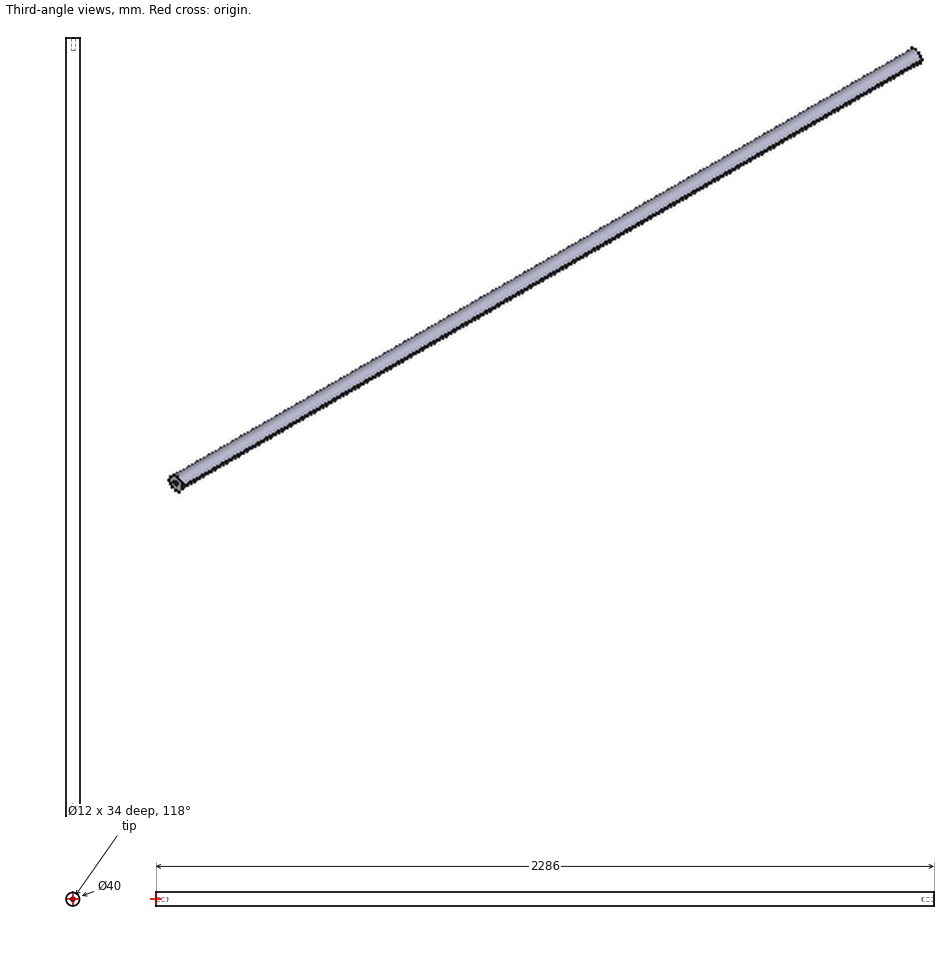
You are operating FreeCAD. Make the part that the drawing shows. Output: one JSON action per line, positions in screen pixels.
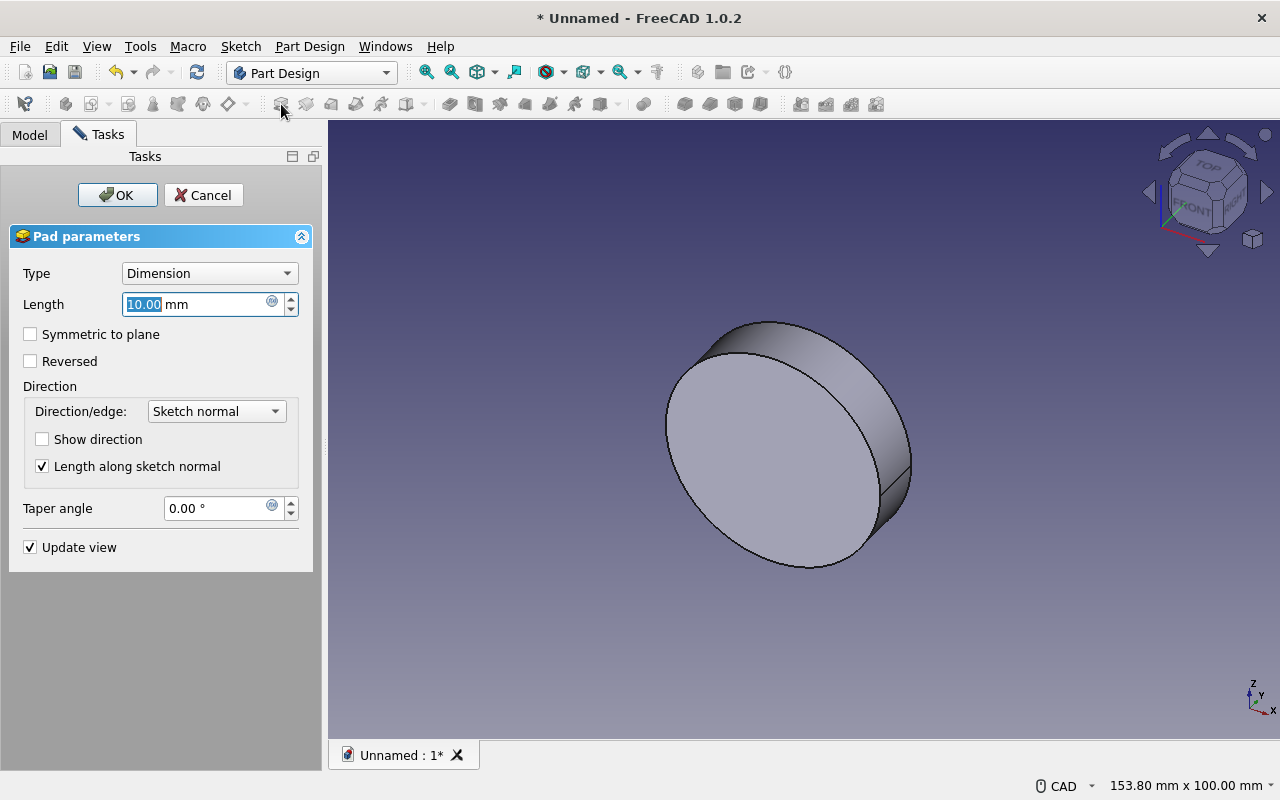
{"action": "type", "text": "2286"}
{"action": "key", "text": "Tab"}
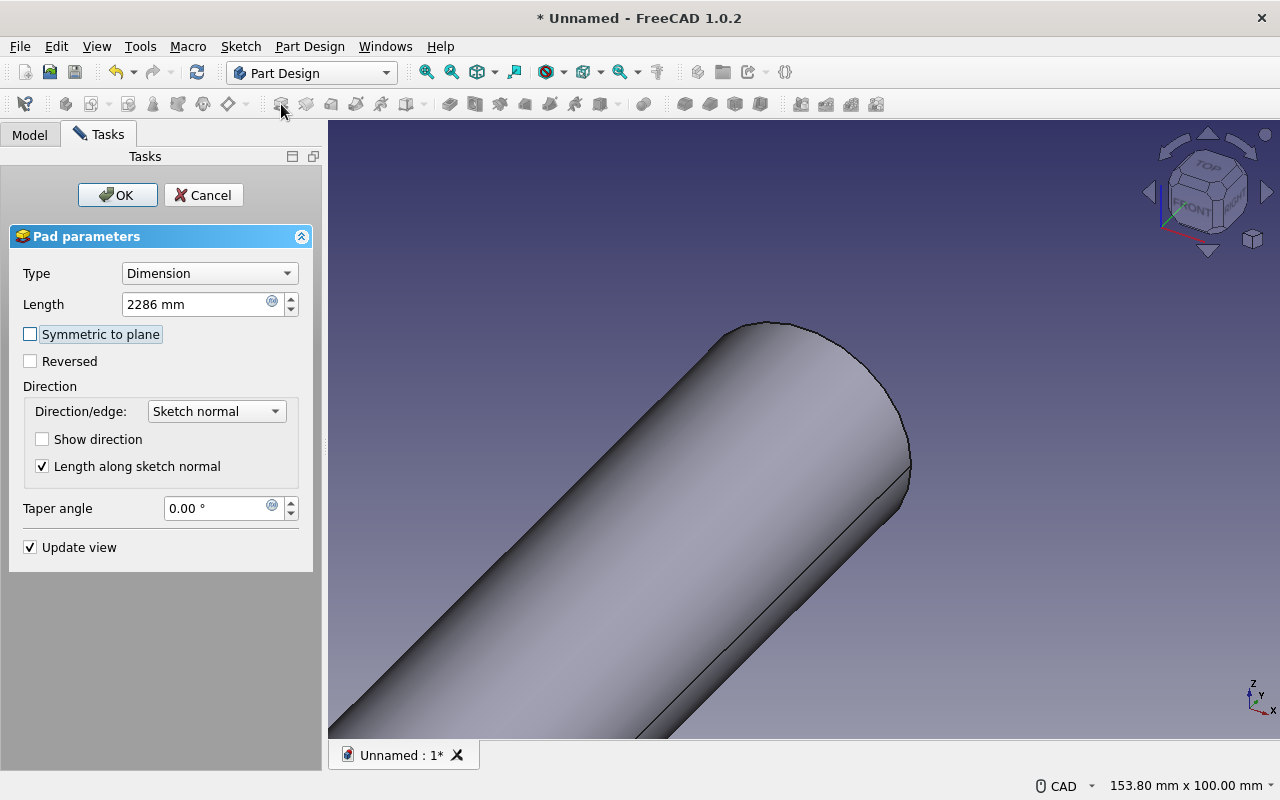
{"action": "left_click", "coordinate": [31, 361]}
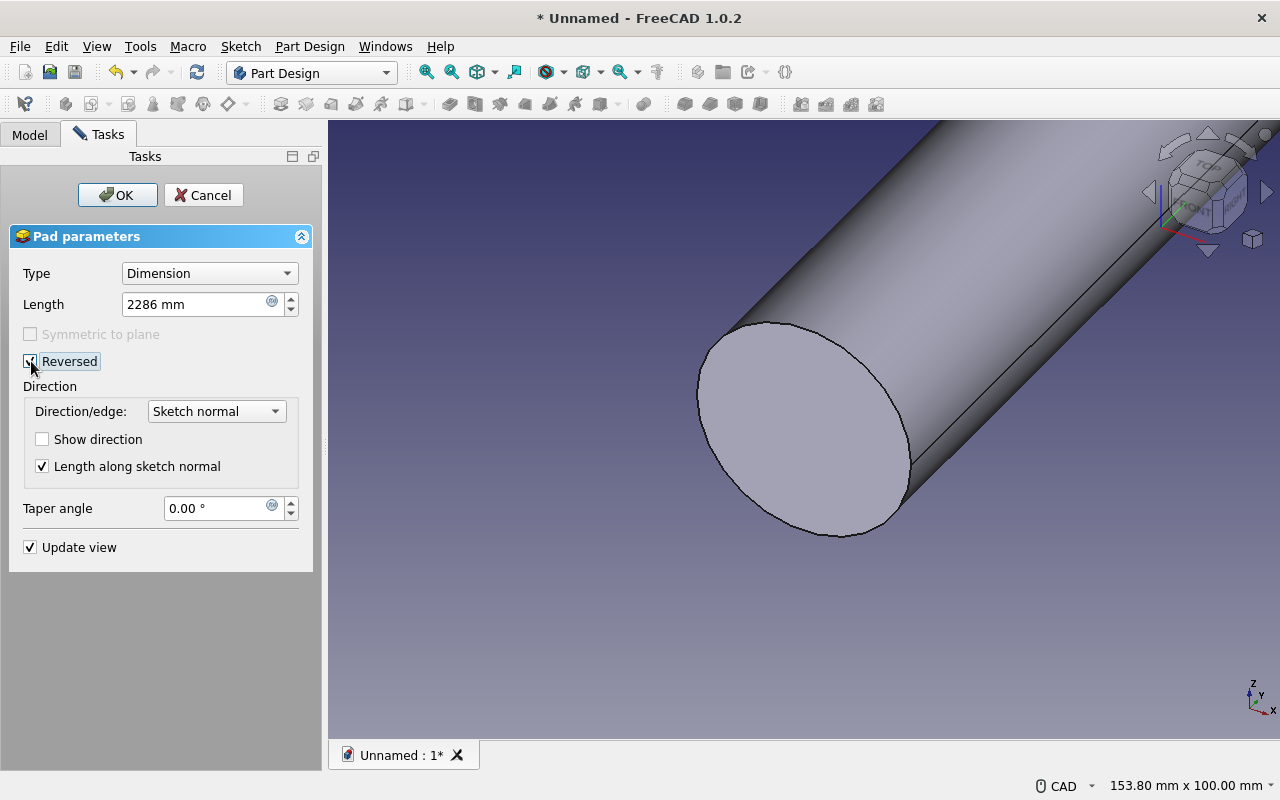
{"action": "left_click", "coordinate": [118, 195]}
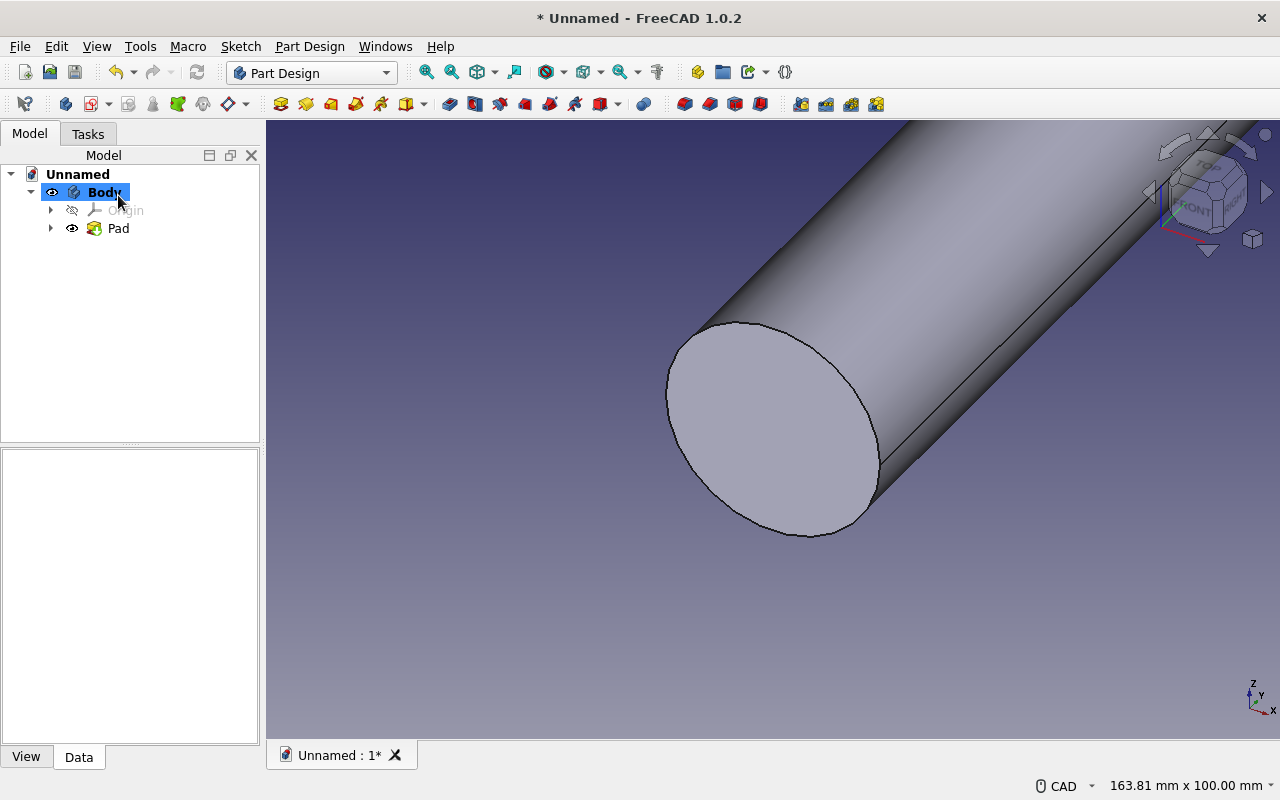
{"action": "left_click", "coordinate": [427, 72]}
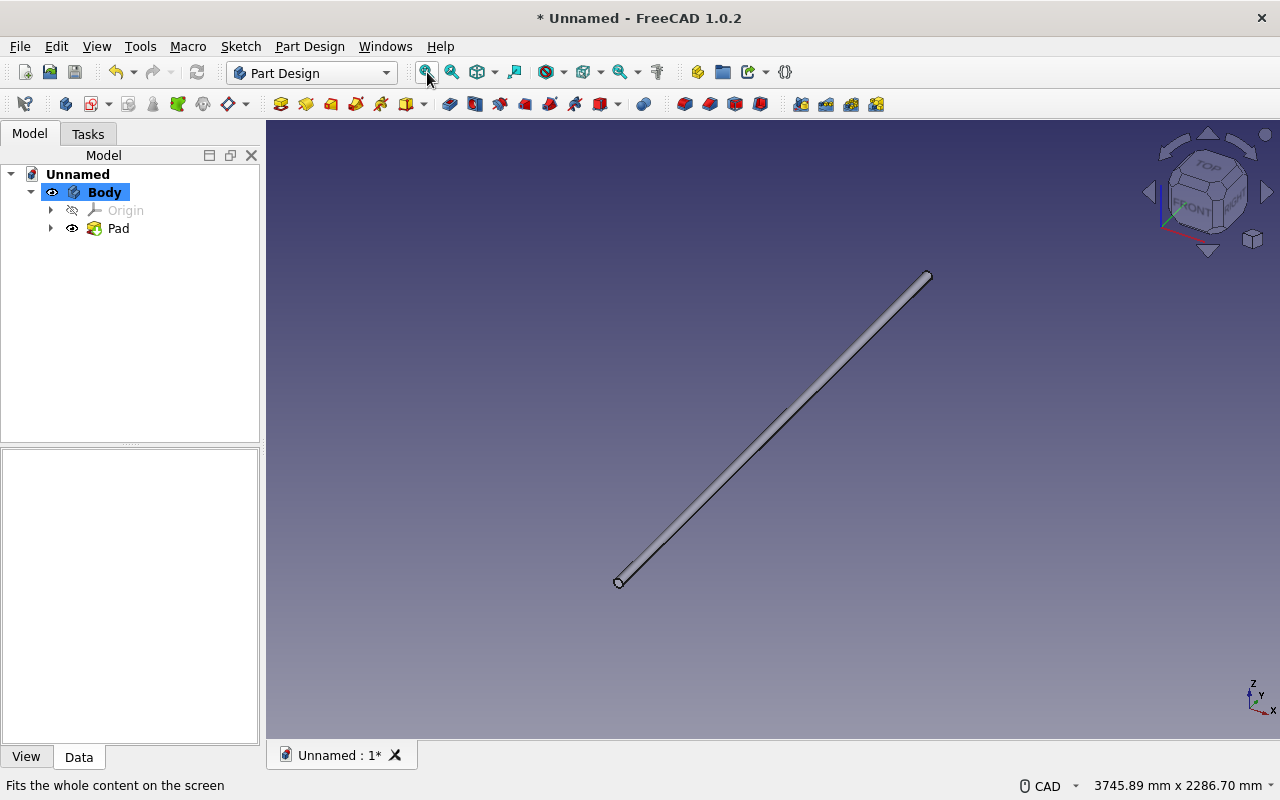
{"action": "key", "text": "4"}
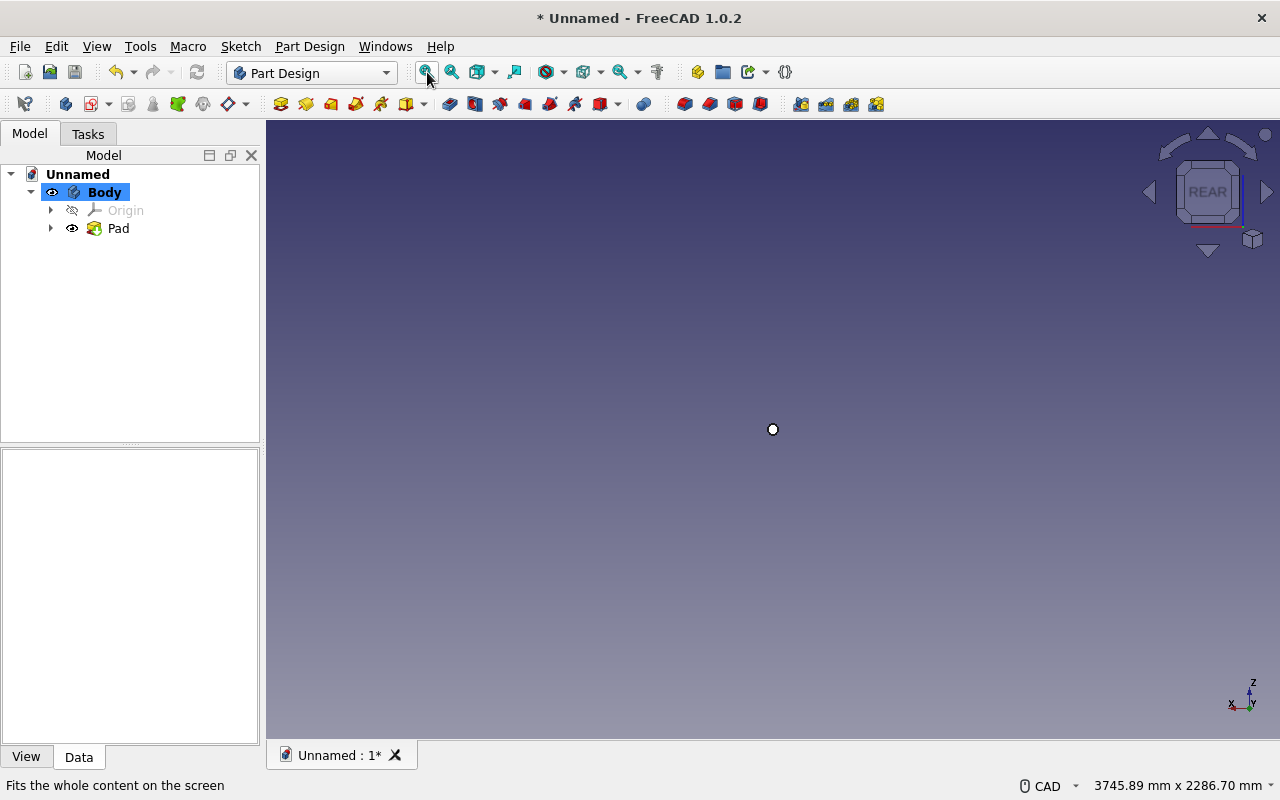
{"action": "left_click", "coordinate": [427, 72]}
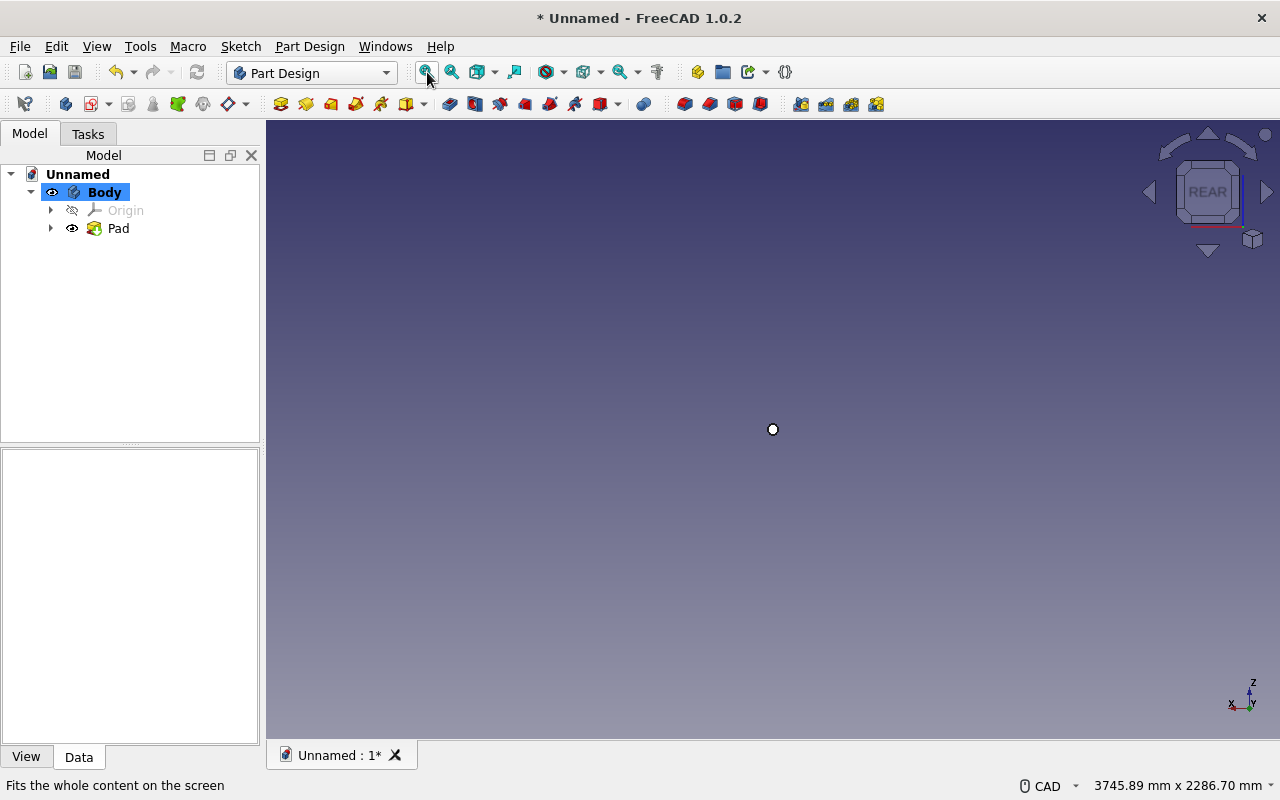
{"action": "scroll", "coordinate": [773, 429], "scroll_direction": "up", "scroll_amount": 4}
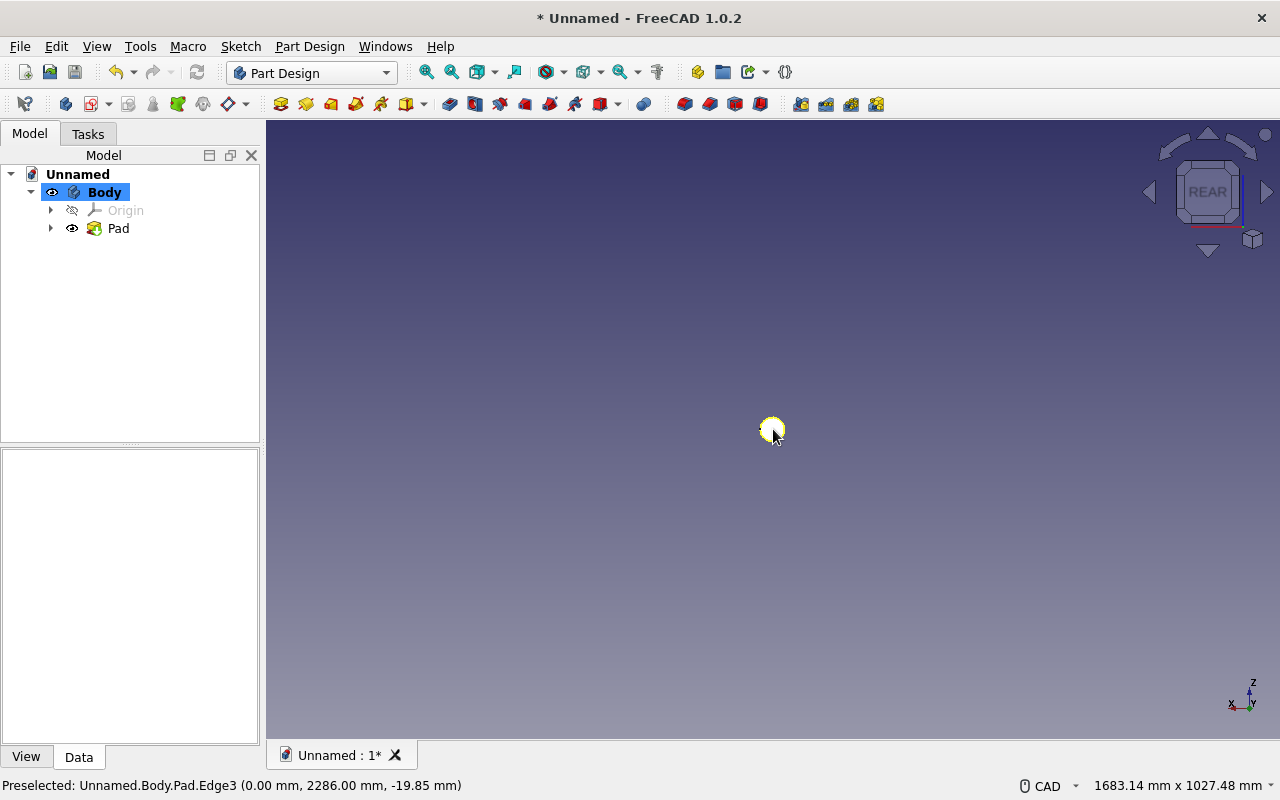
{"action": "left_click", "coordinate": [772, 429]}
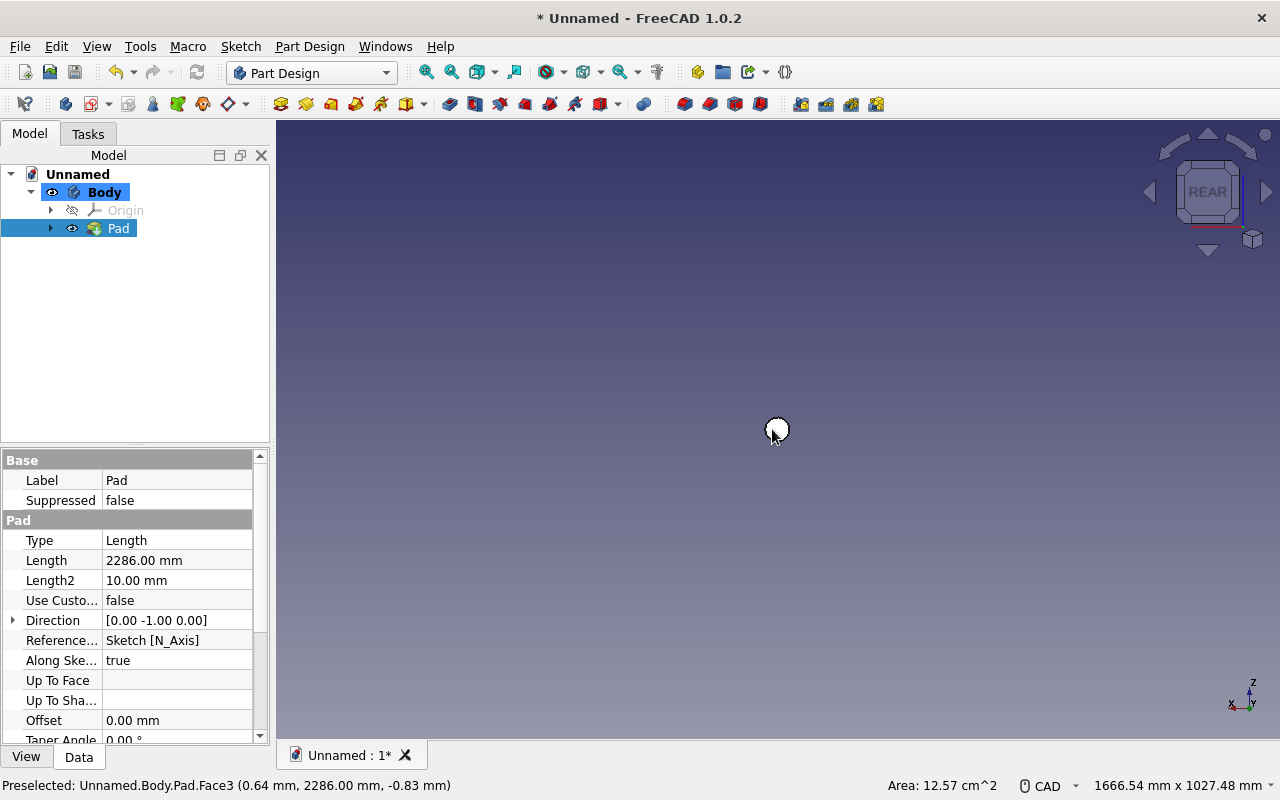
{"action": "left_click", "coordinate": [90, 104]}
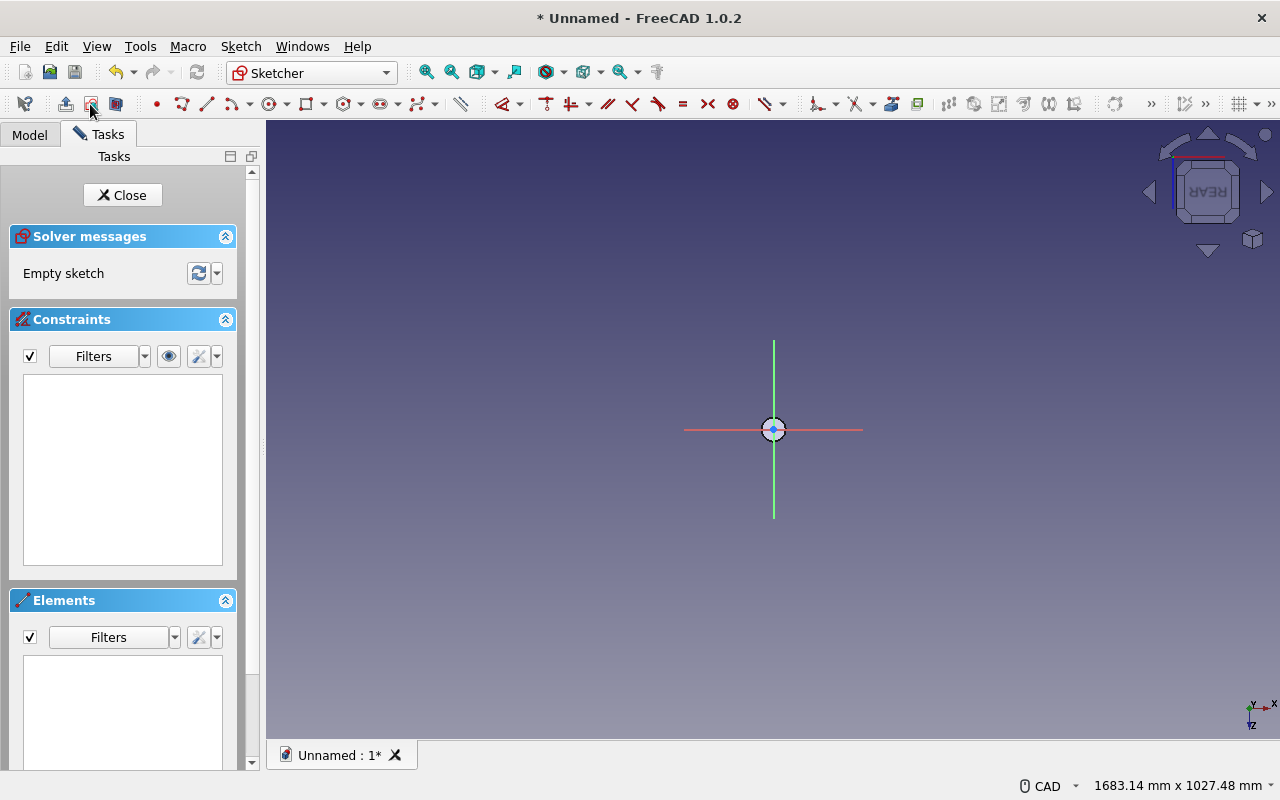
{"action": "scroll", "coordinate": [777, 429], "scroll_direction": "up", "scroll_amount": 15}